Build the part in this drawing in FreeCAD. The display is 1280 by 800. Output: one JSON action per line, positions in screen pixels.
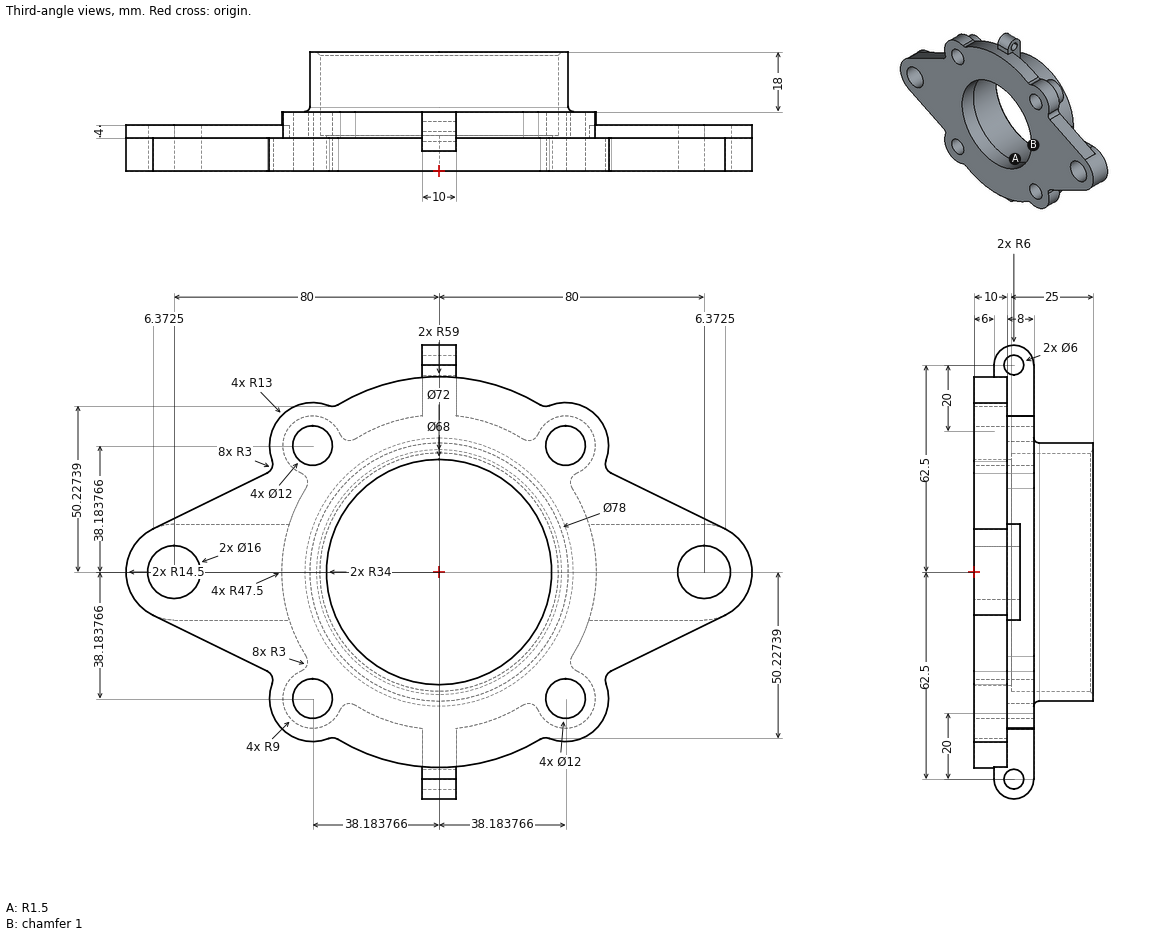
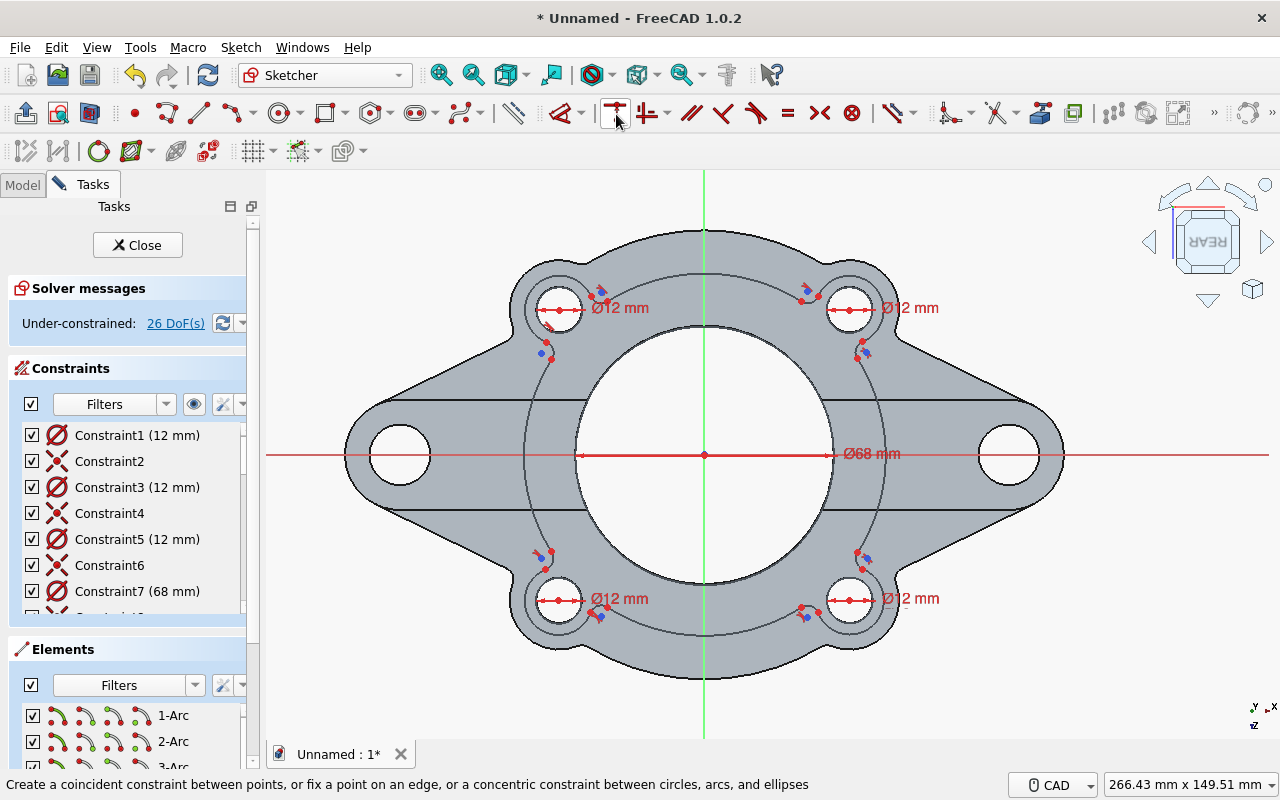
{"action": "scroll", "coordinate": [705, 455], "scroll_direction": "up", "scroll_amount": 7}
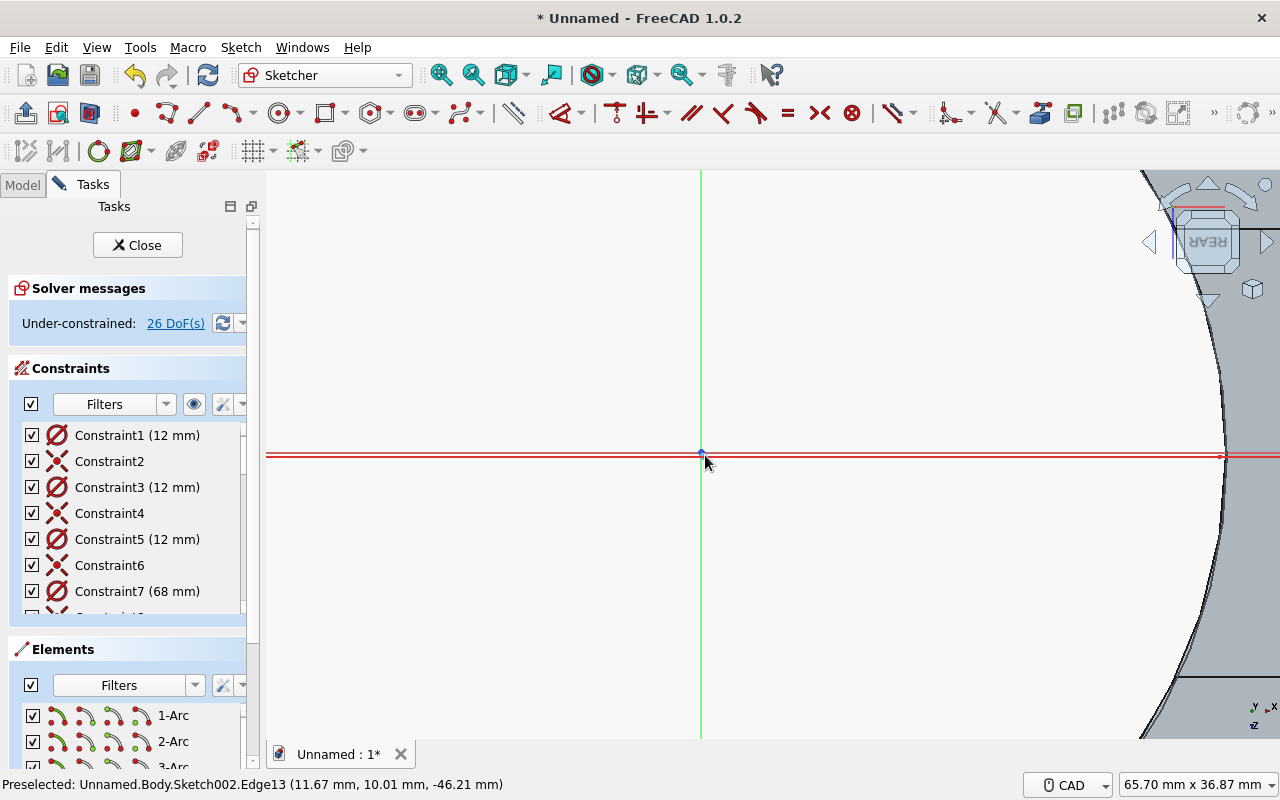
{"action": "left_click_drag", "start_coordinate": [691, 443], "coordinate": [712, 467]}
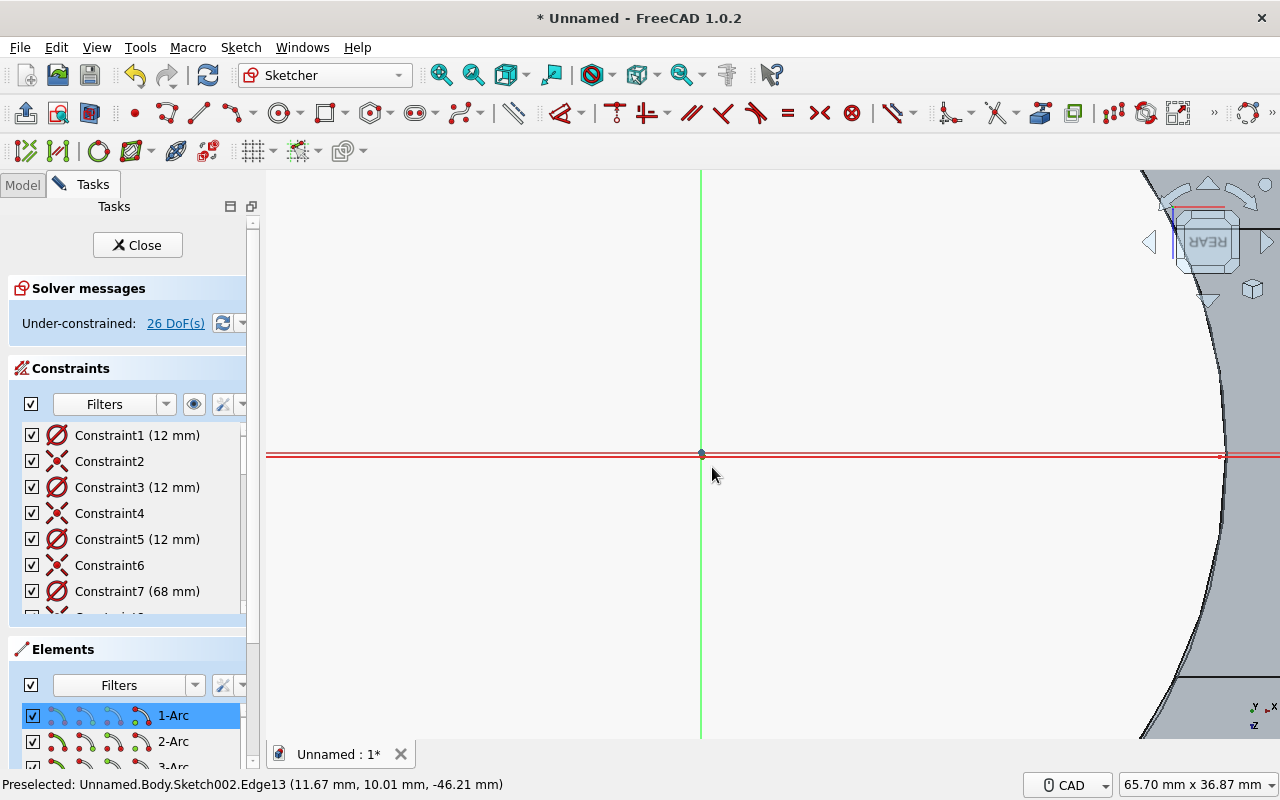
{"action": "left_click", "coordinate": [616, 114]}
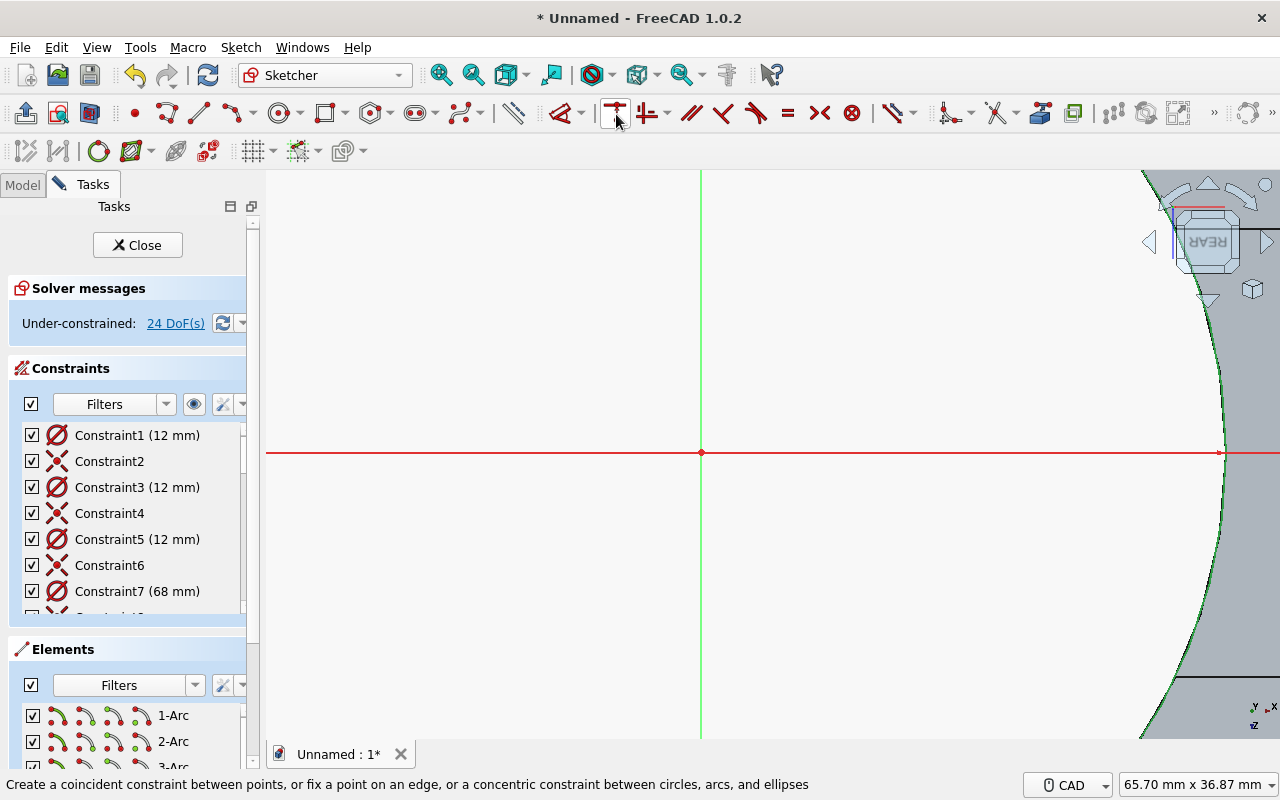
{"action": "scroll", "coordinate": [706, 455], "scroll_direction": "down", "scroll_amount": 7}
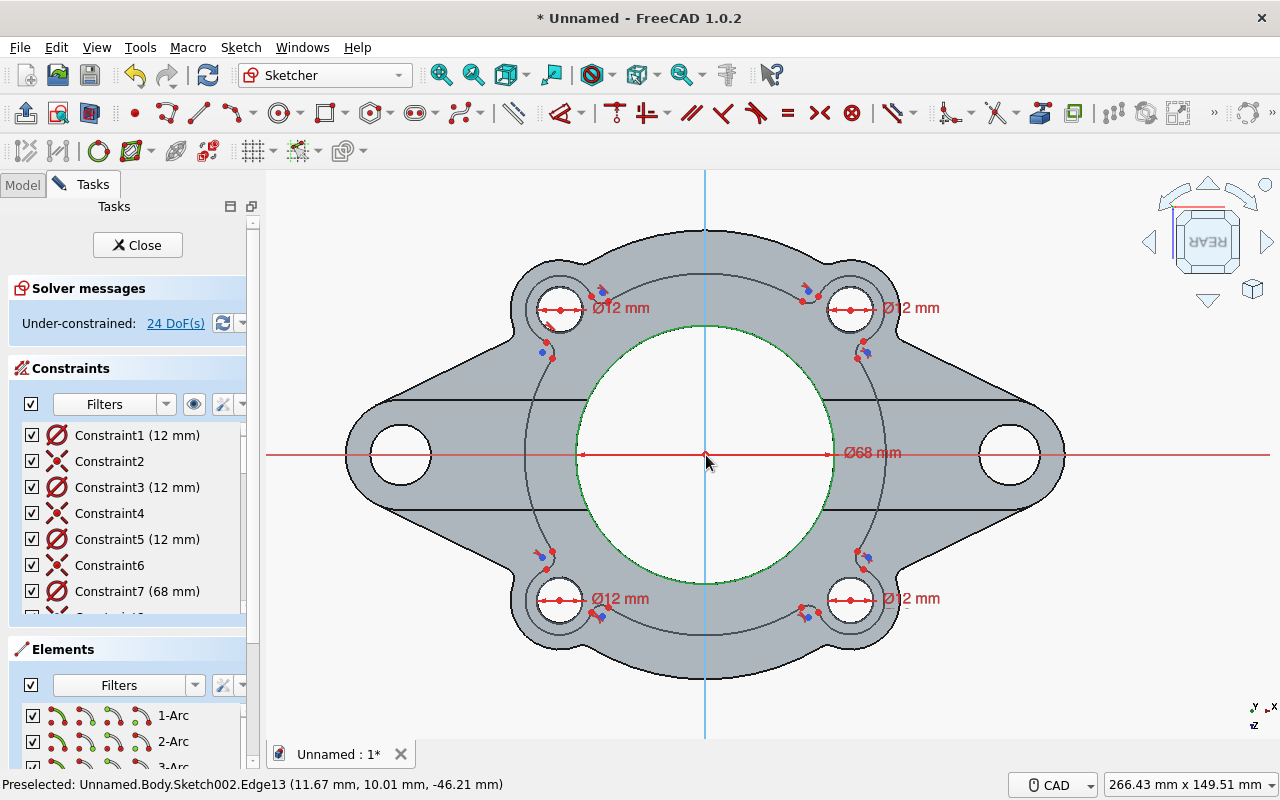
{"action": "scroll", "coordinate": [552, 566], "scroll_direction": "up", "scroll_amount": 4}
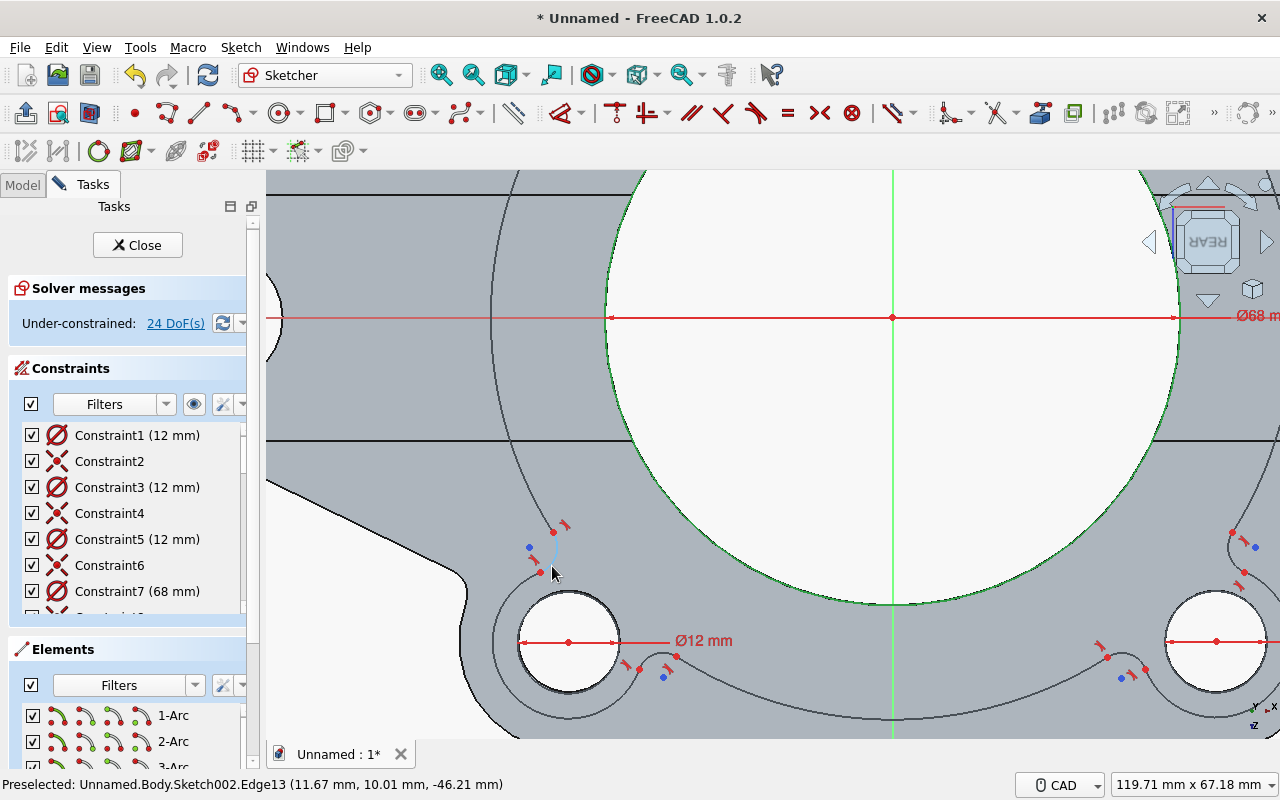
{"action": "left_click", "coordinate": [551, 564]}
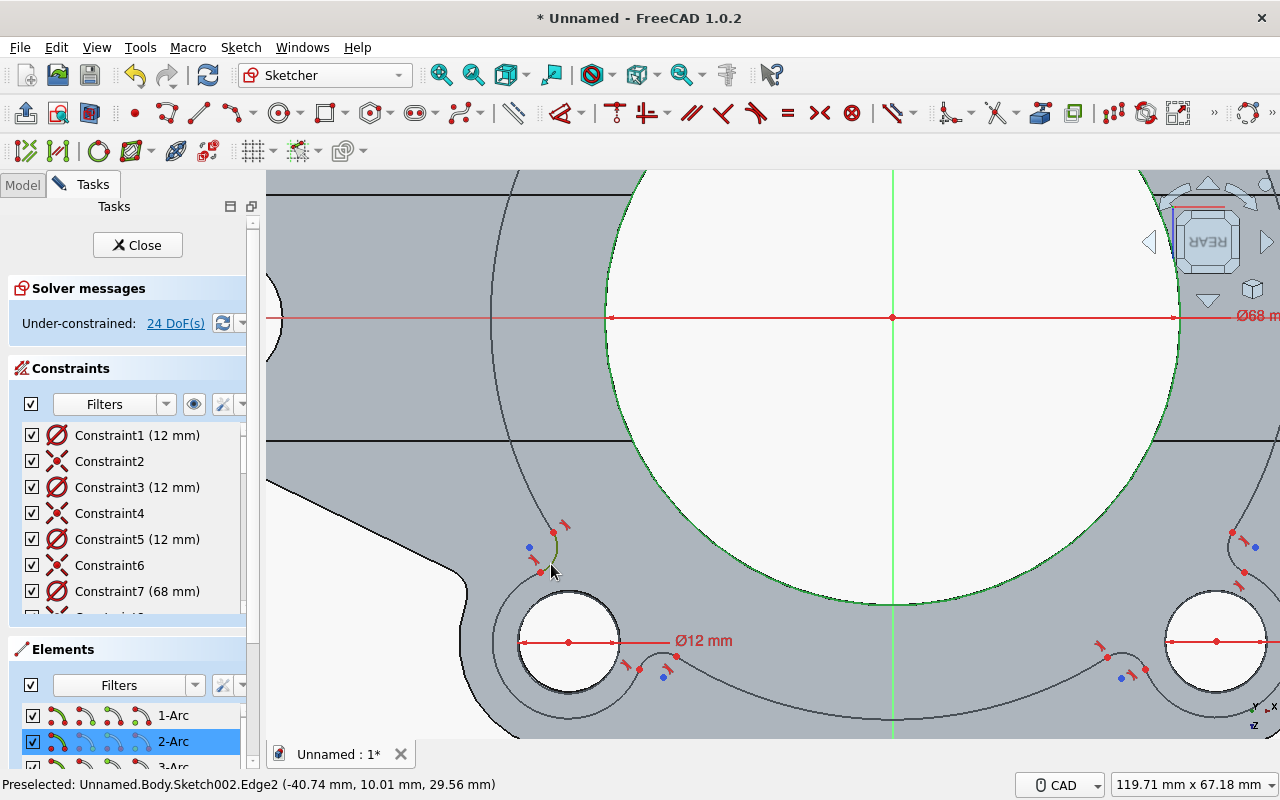
{"action": "left_click", "coordinate": [664, 653]}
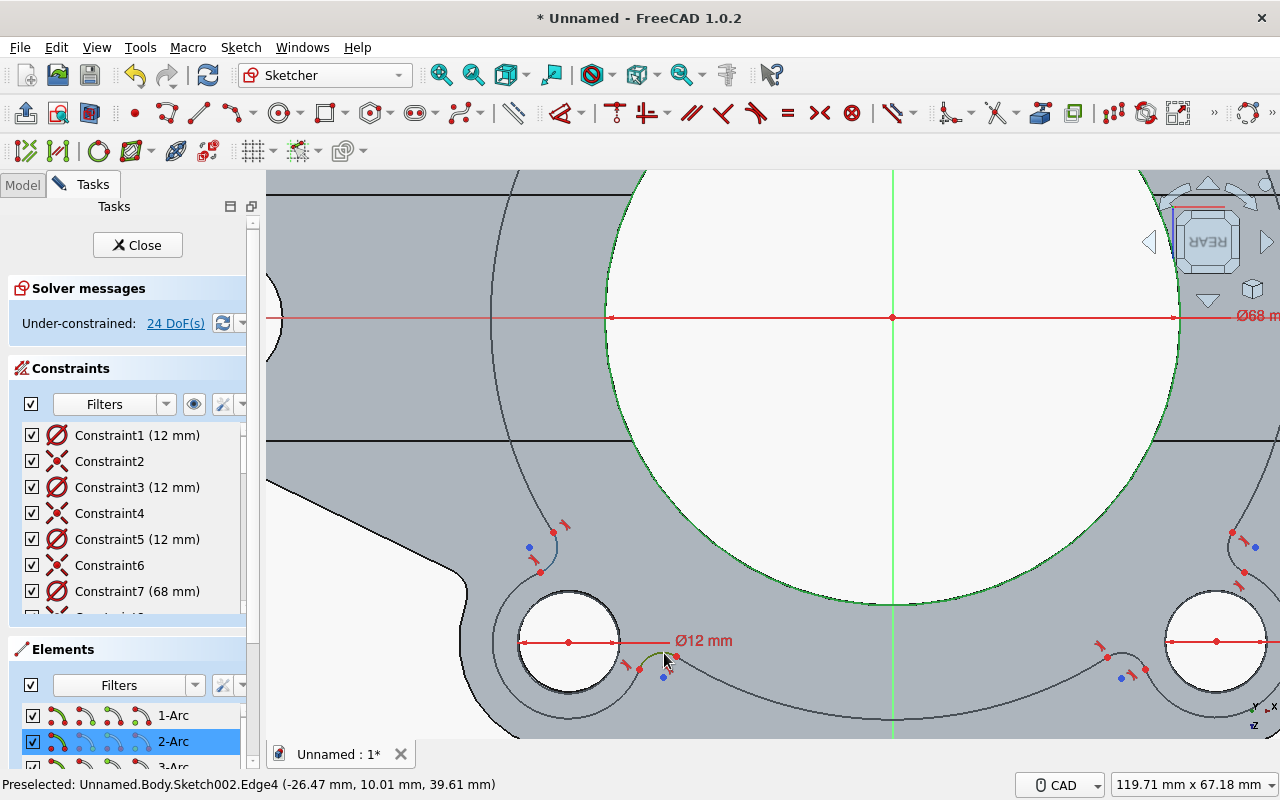
{"action": "scroll", "coordinate": [551, 566], "scroll_direction": "down", "scroll_amount": 4}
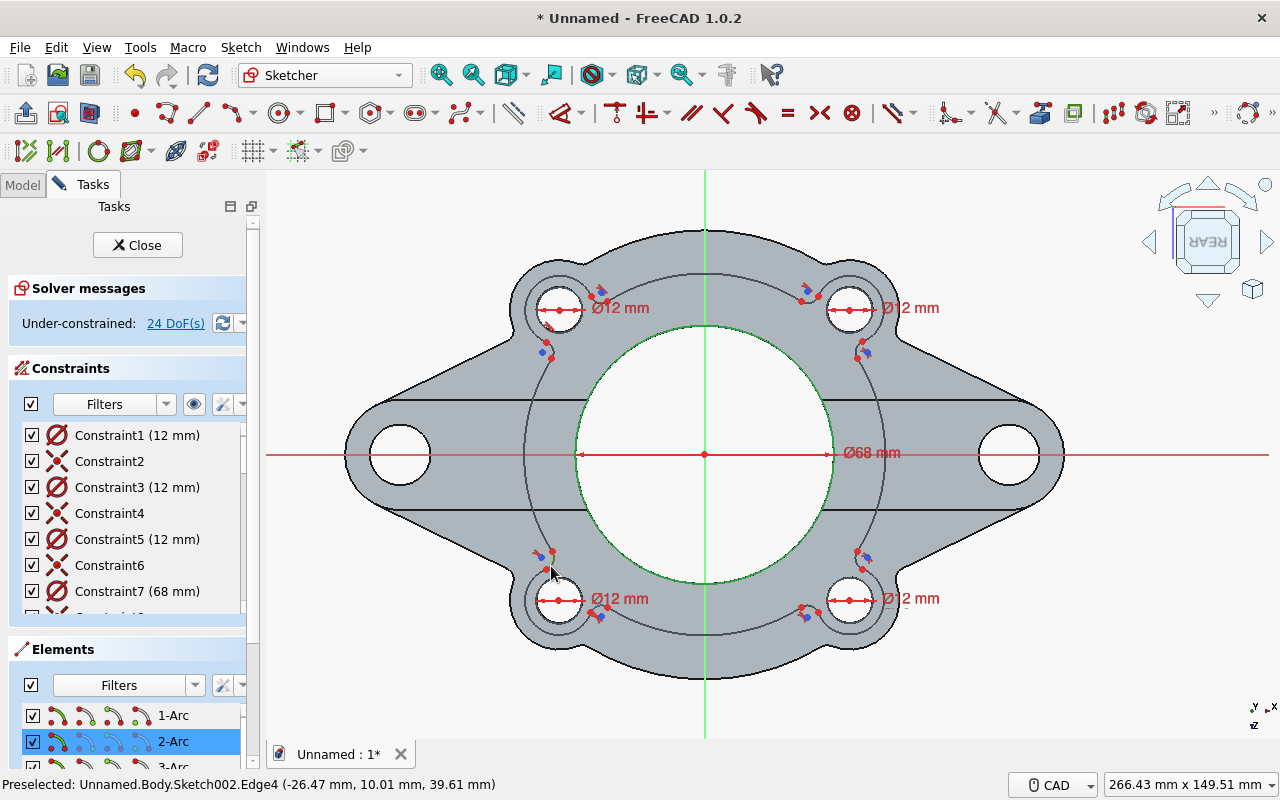
{"action": "scroll", "coordinate": [815, 608], "scroll_direction": "up", "scroll_amount": 5}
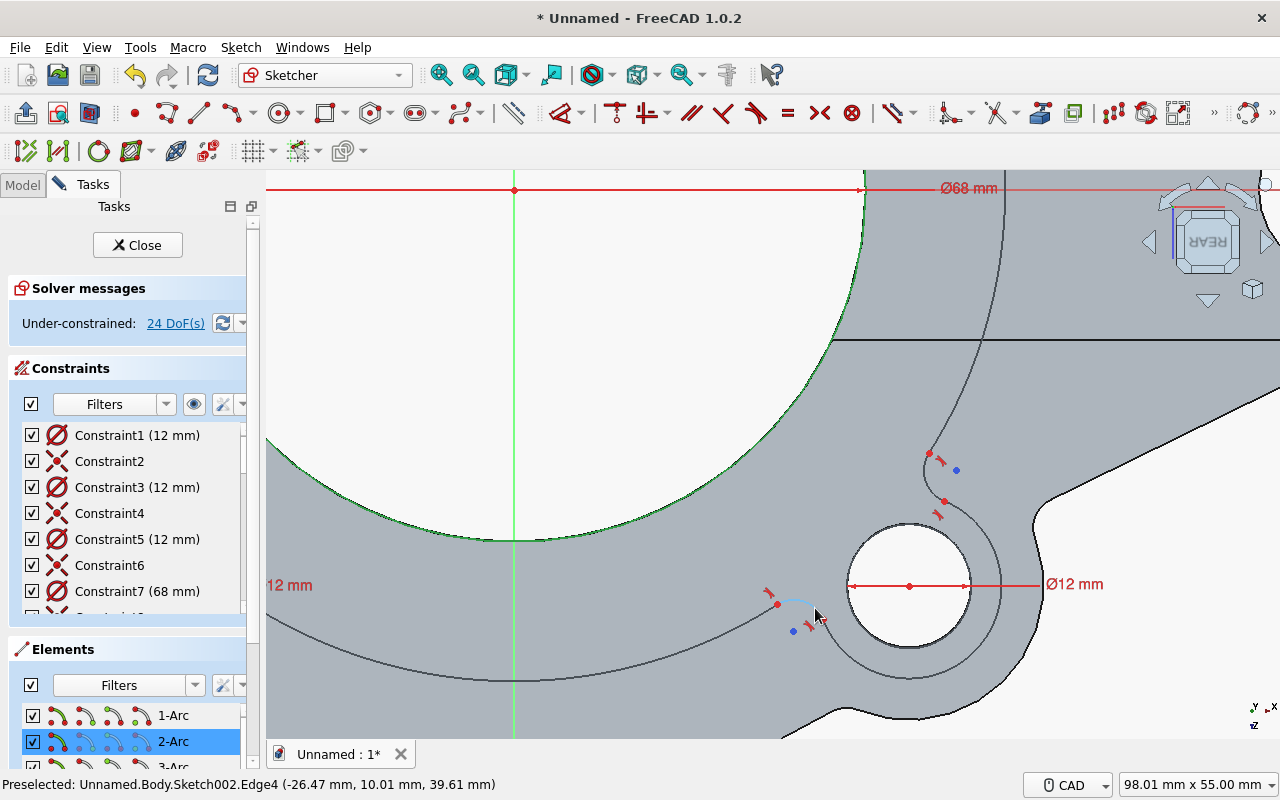
{"action": "left_click", "coordinate": [813, 607]}